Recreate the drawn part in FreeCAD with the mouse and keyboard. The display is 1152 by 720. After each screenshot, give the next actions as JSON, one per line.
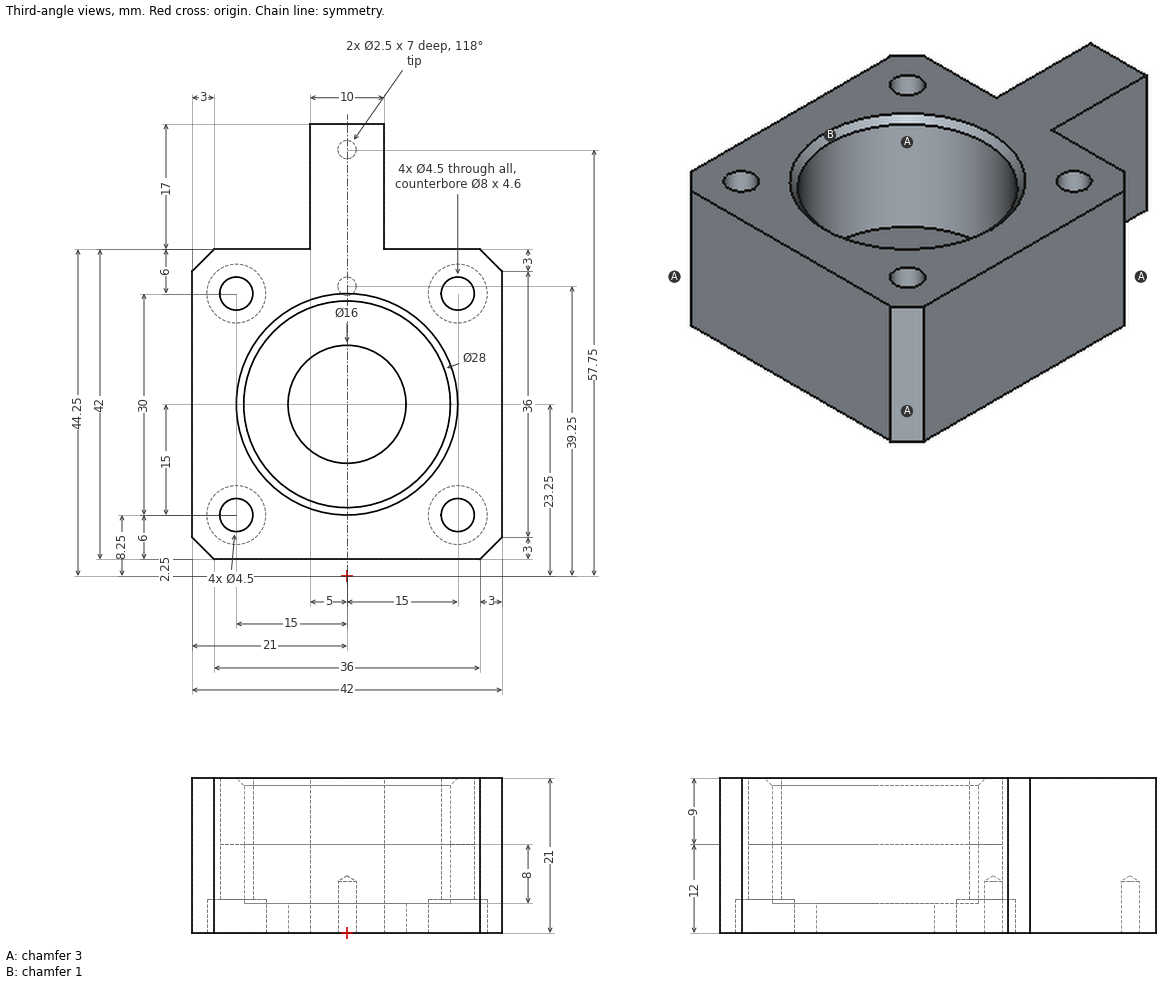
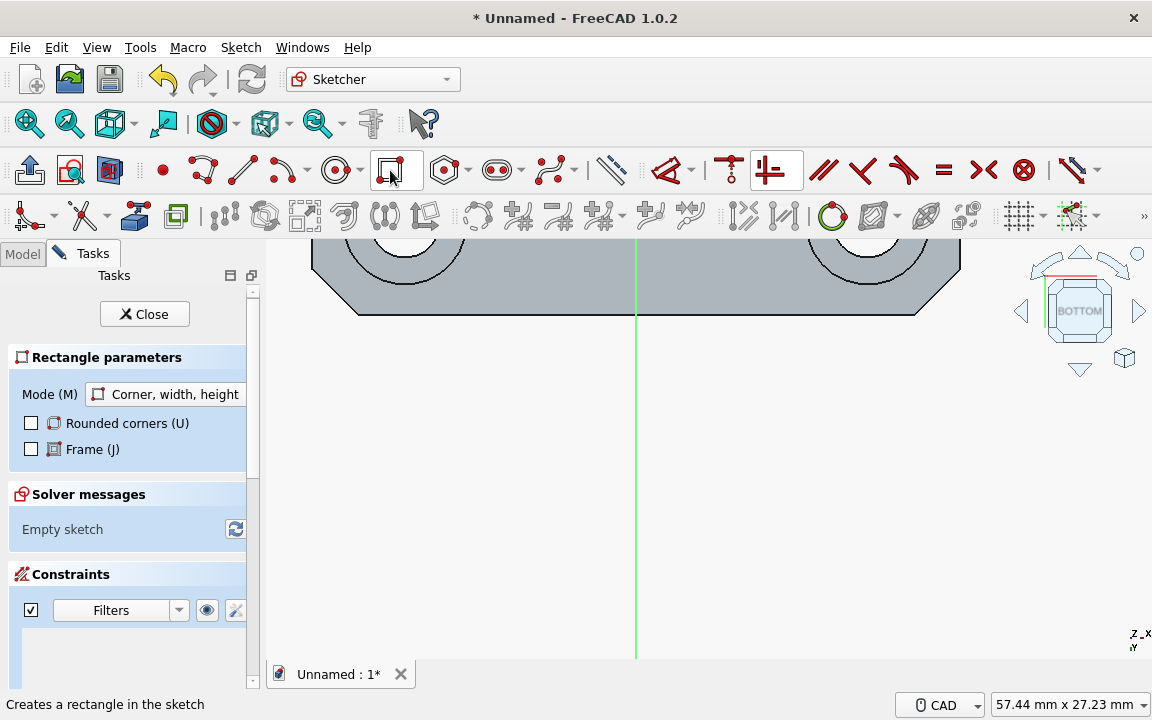
{"action": "left_click", "coordinate": [559, 315]}
{"action": "left_click", "coordinate": [713, 578]}
{"action": "key", "text": "Escape"}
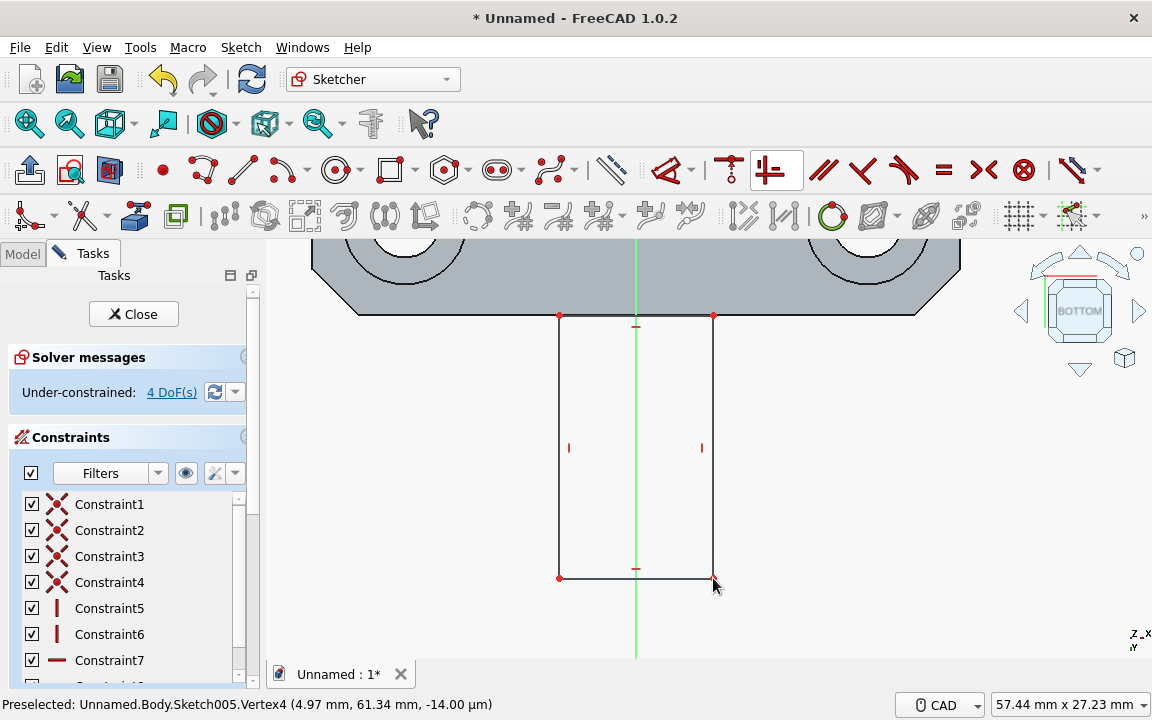
{"action": "left_click", "coordinate": [666, 170]}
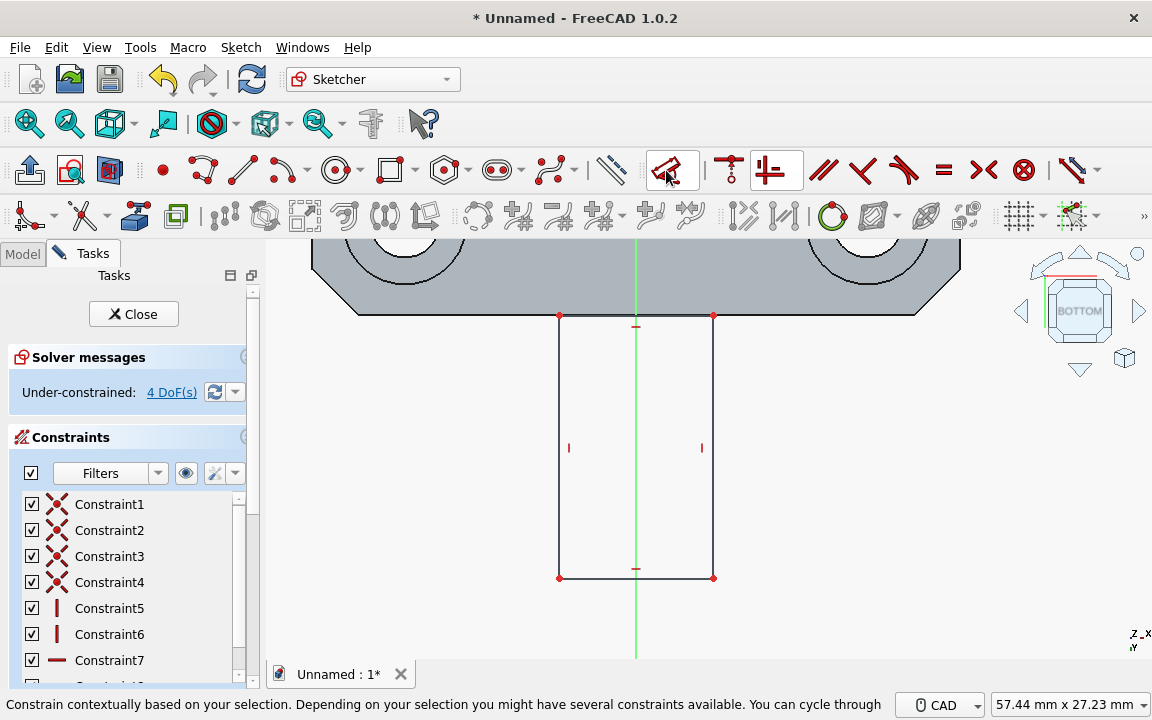
{"action": "left_click", "coordinate": [559, 395]}
{"action": "left_click", "coordinate": [525, 448]}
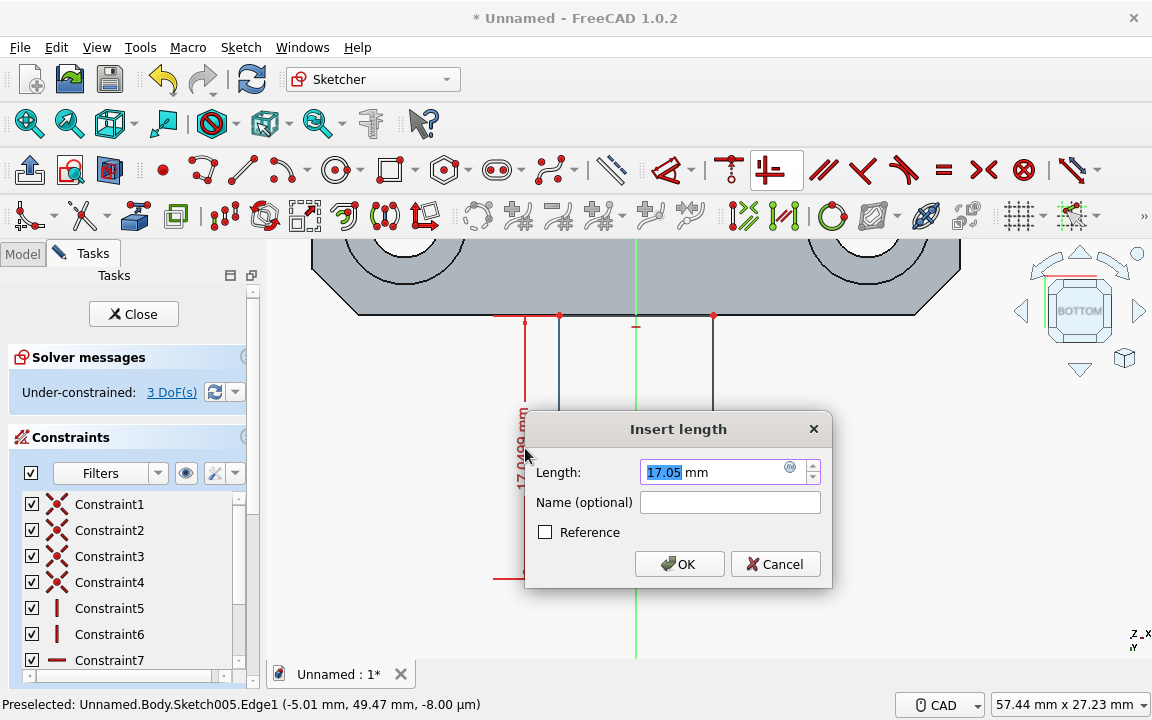
{"action": "type", "text": "17"}
{"action": "key", "text": "Return"}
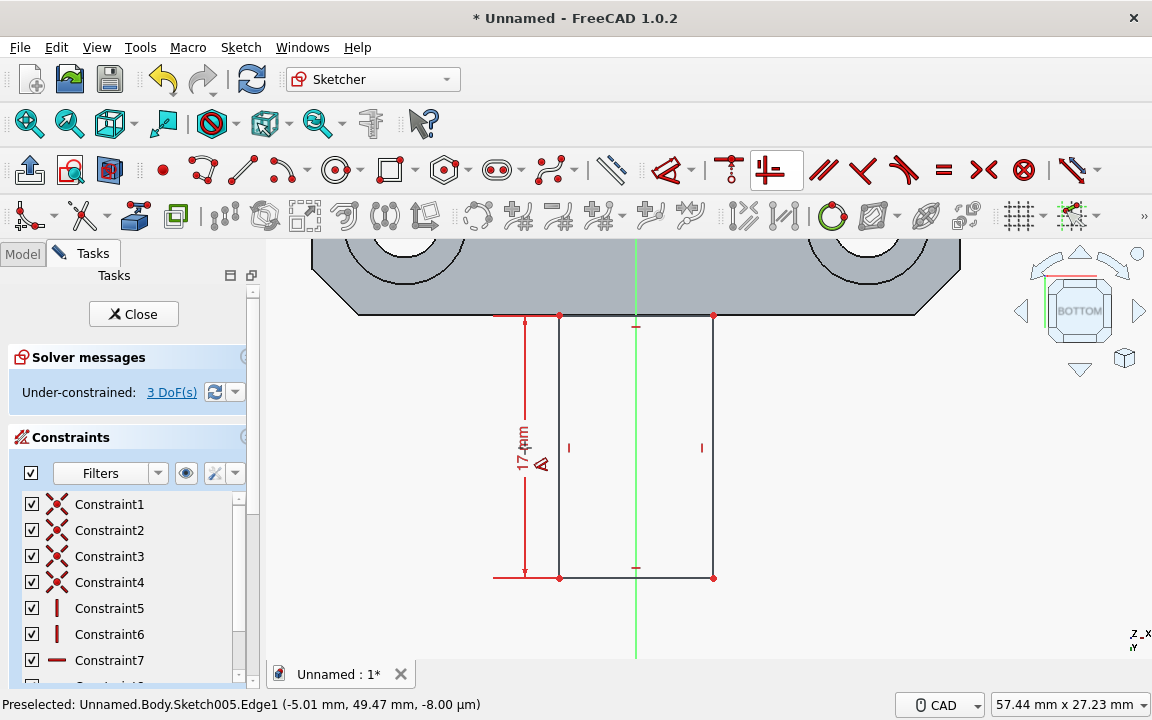
{"action": "left_click", "coordinate": [605, 578]}
{"action": "left_click", "coordinate": [601, 612]}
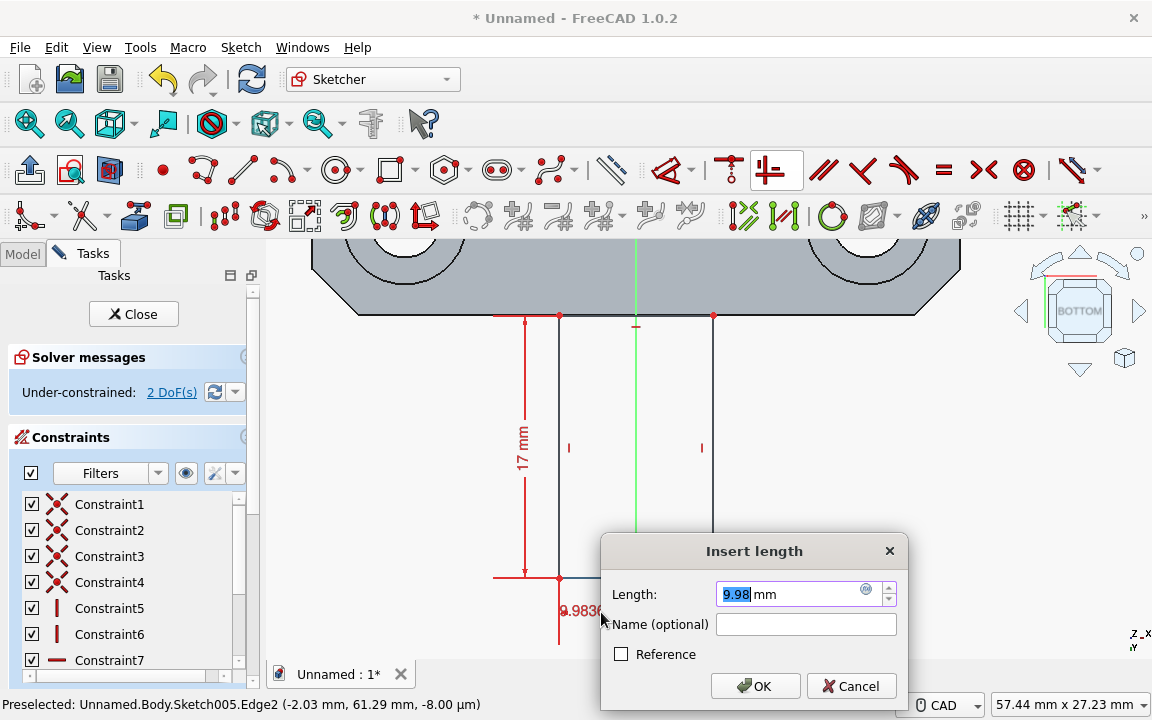
{"action": "type", "text": "10"}
{"action": "key", "text": "Return"}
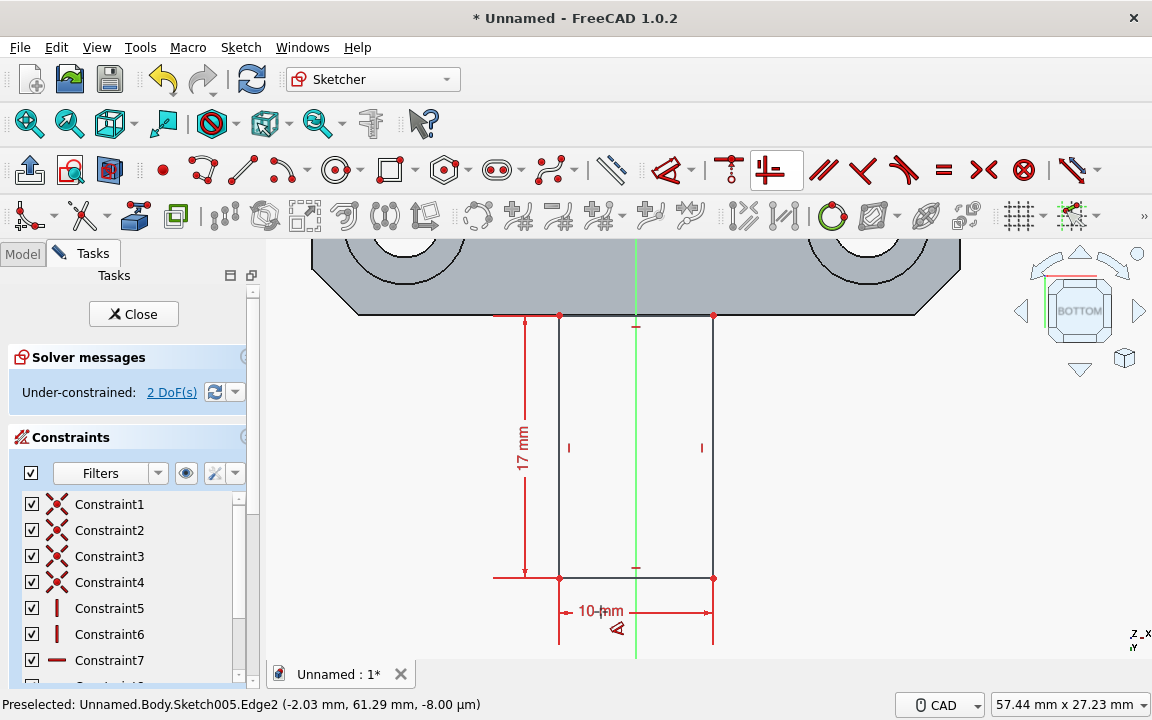
{"action": "left_click", "coordinate": [559, 316]}
{"action": "left_click", "coordinate": [598, 350]}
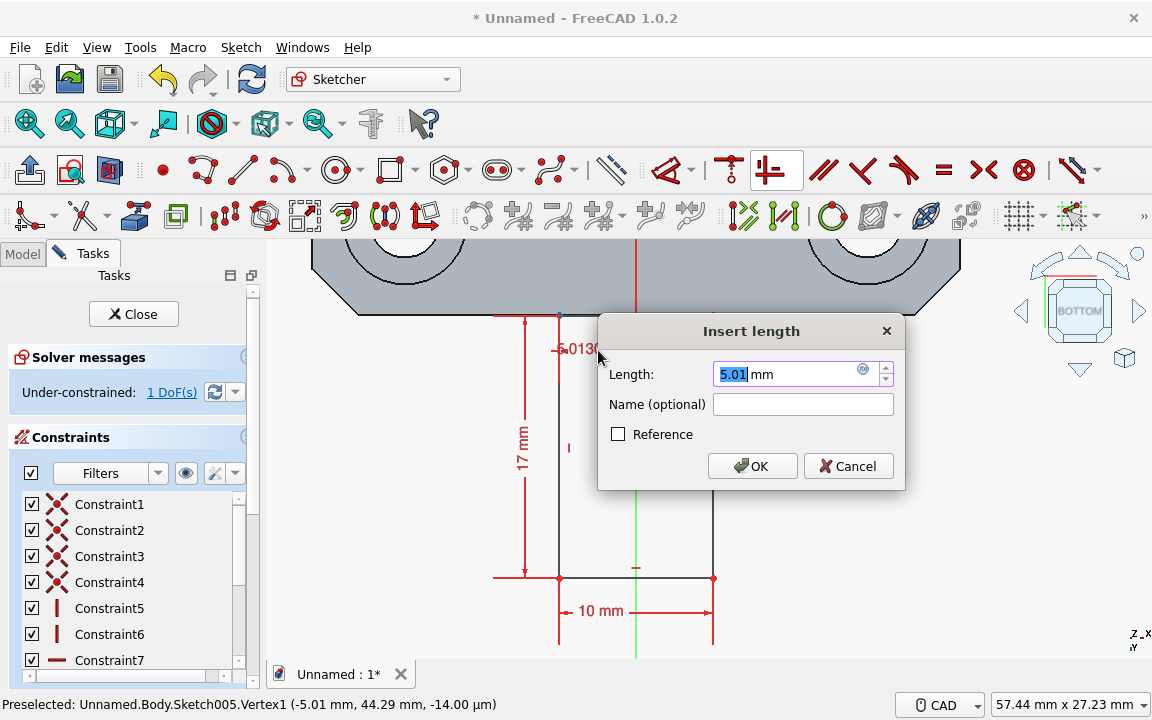
{"action": "type", "text": "5"}
{"action": "key", "text": "Return"}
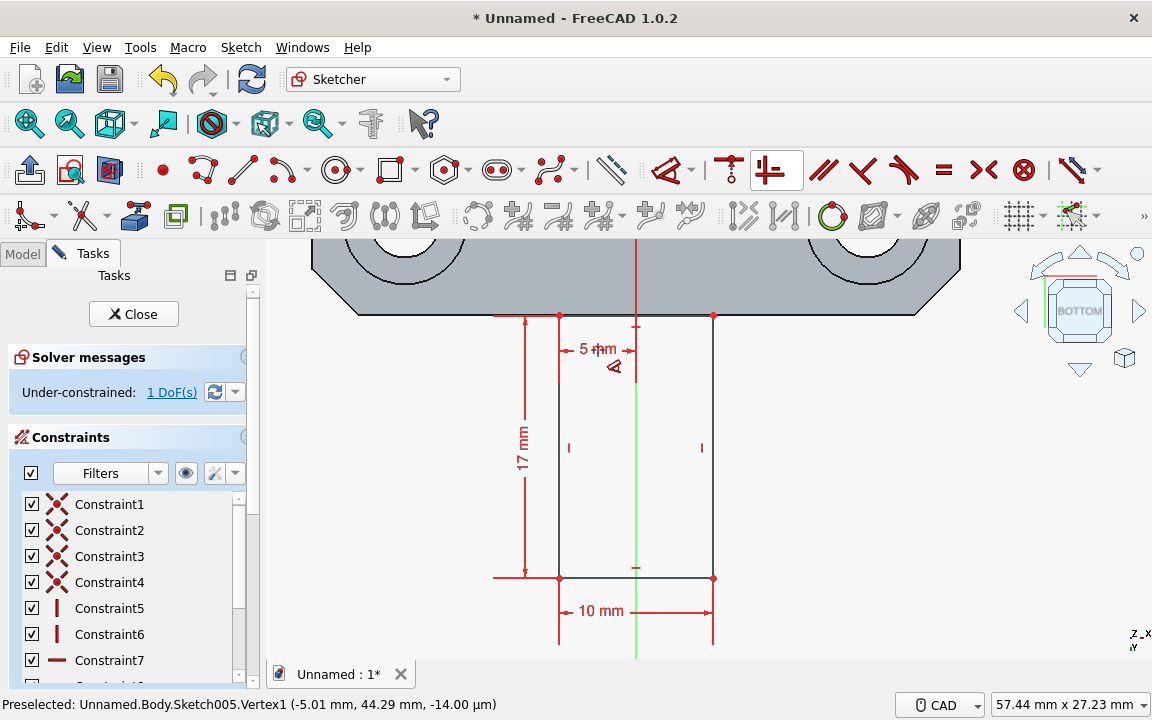
{"action": "left_click", "coordinate": [559, 316]}
{"action": "left_click", "coordinate": [525, 291]}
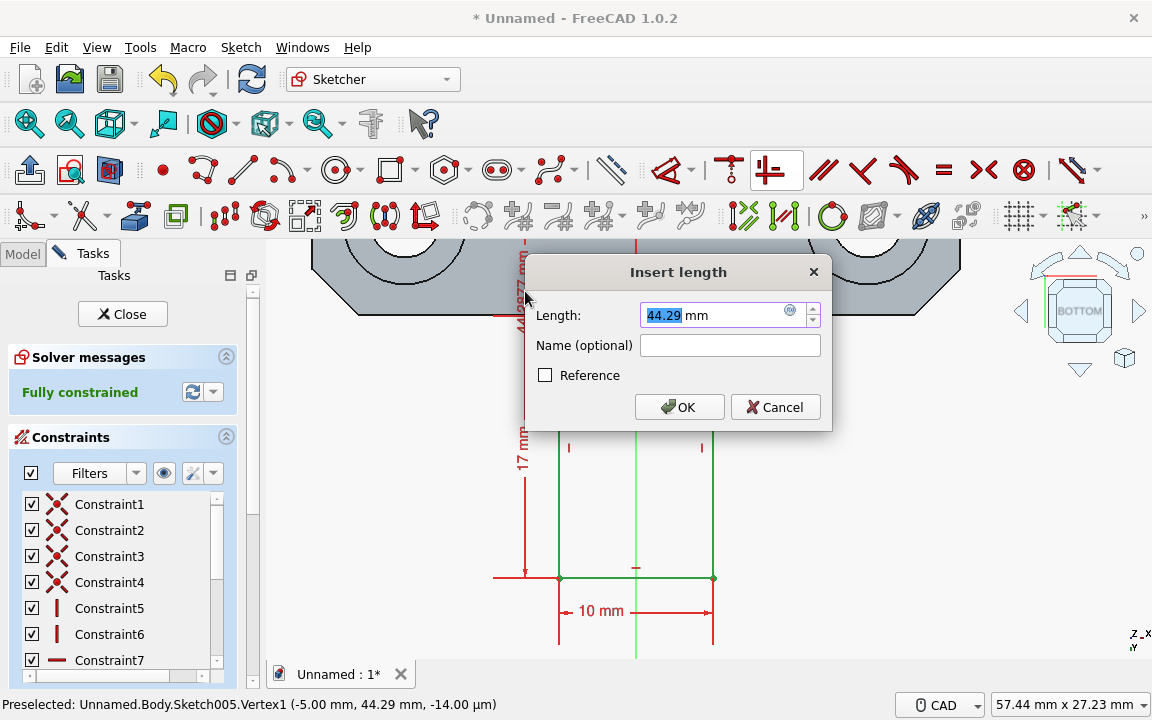
{"action": "type", "text": "44.25"}
{"action": "key", "text": "Return"}
{"action": "key", "text": "Escape"}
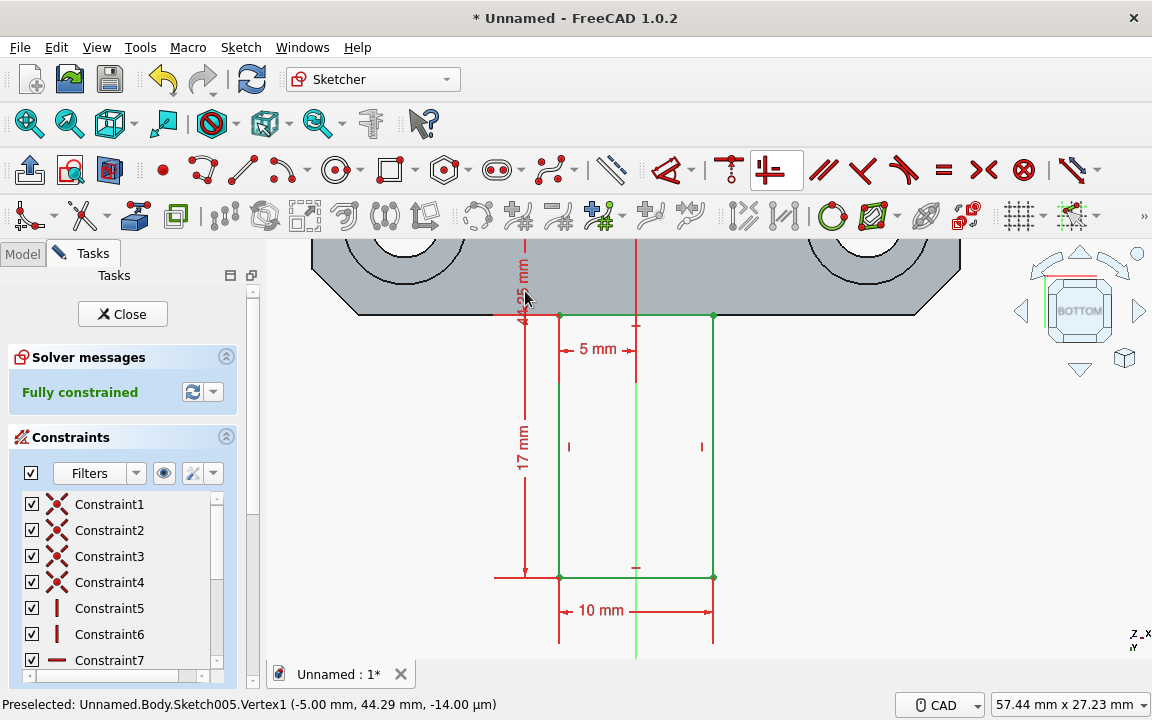
{"action": "left_click", "coordinate": [123, 314]}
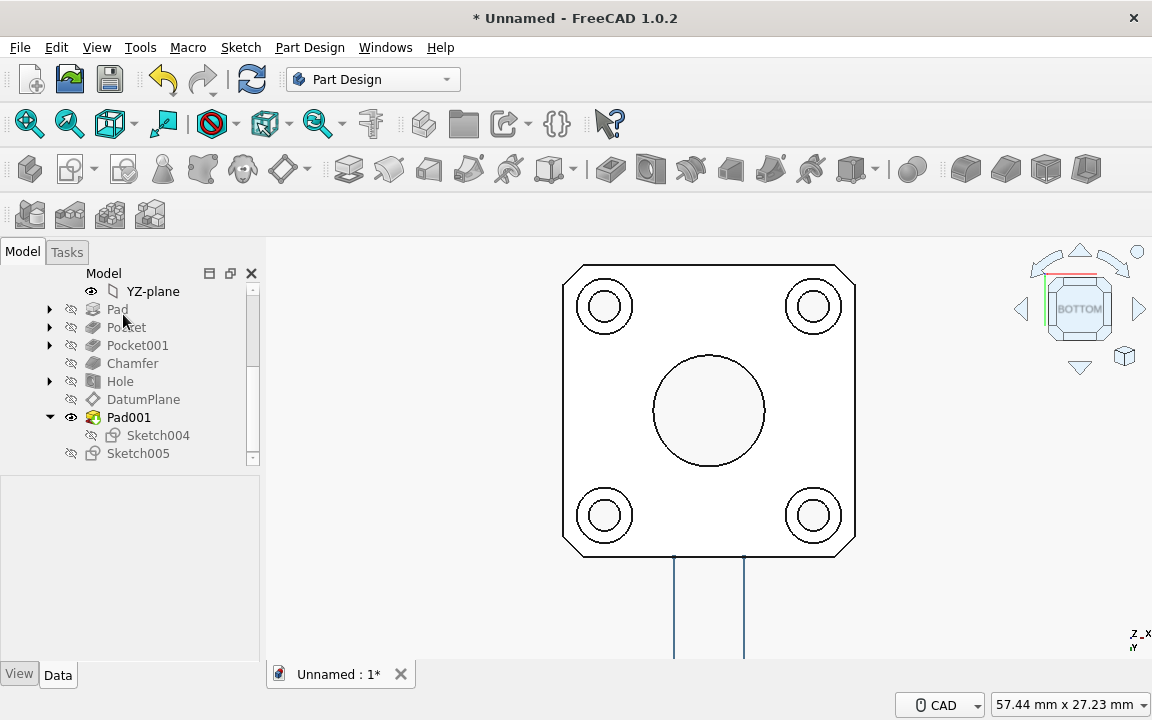
{"action": "left_click", "coordinate": [350, 170]}